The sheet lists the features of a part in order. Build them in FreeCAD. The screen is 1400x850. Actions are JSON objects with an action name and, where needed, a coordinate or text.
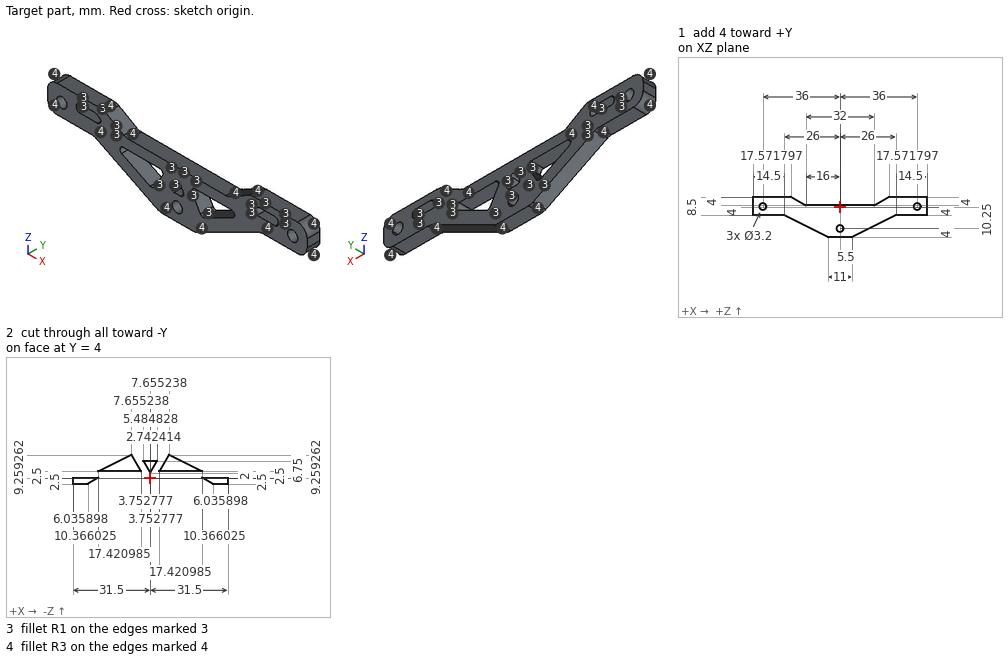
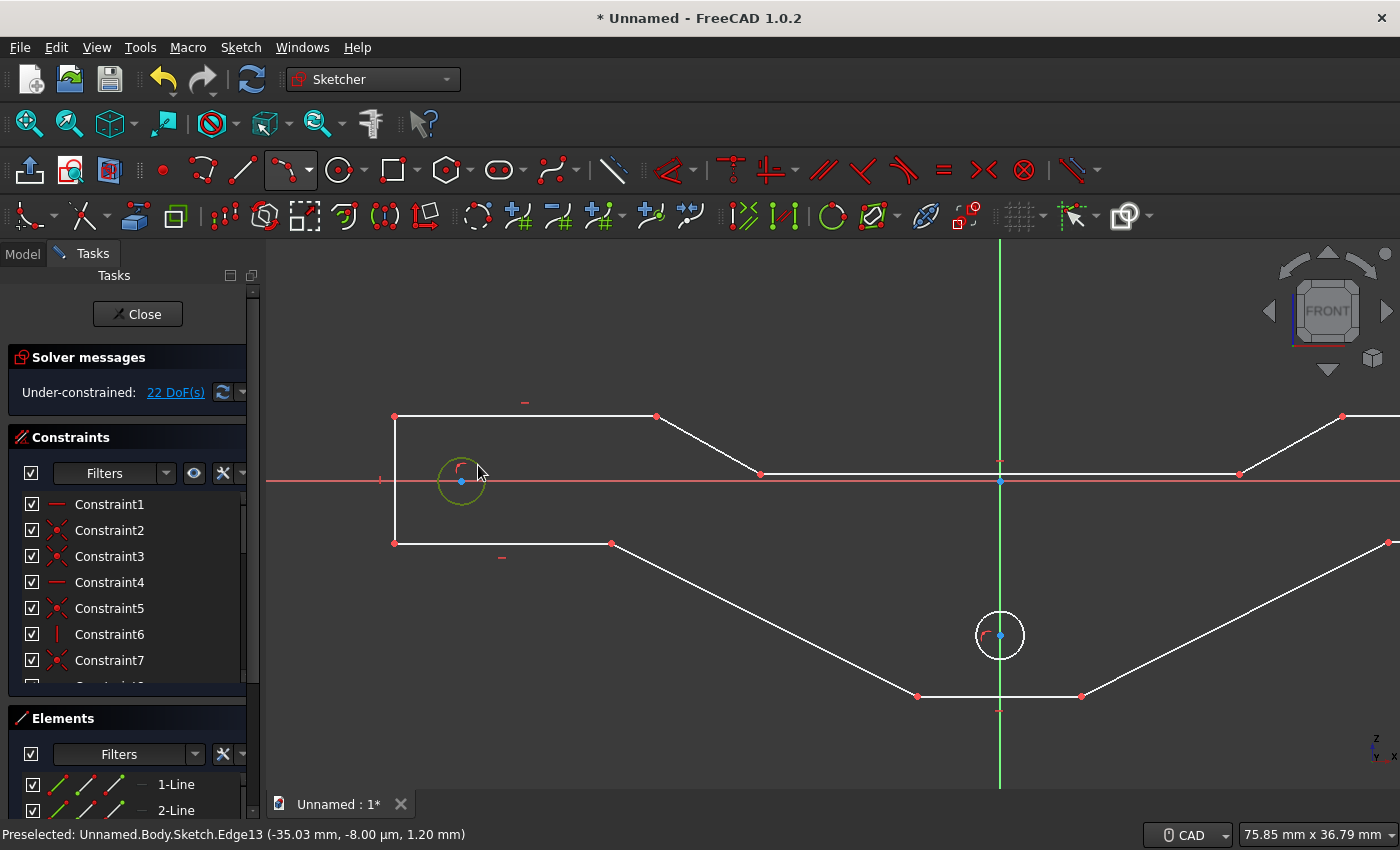
{"action": "scroll", "coordinate": [478, 465], "scroll_direction": "down", "scroll_amount": 3}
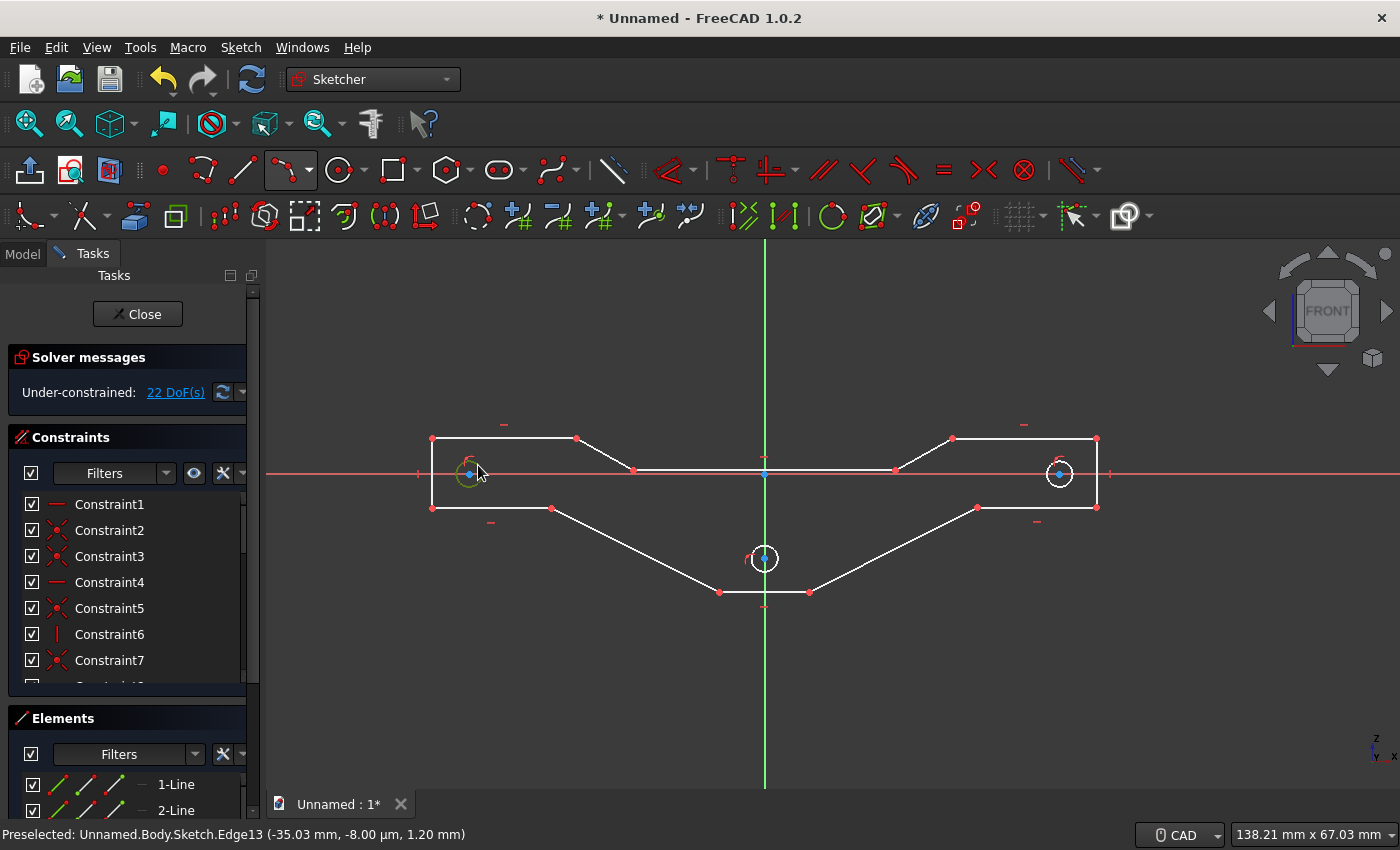
{"action": "scroll", "coordinate": [1069, 465], "scroll_direction": "up", "scroll_amount": 3}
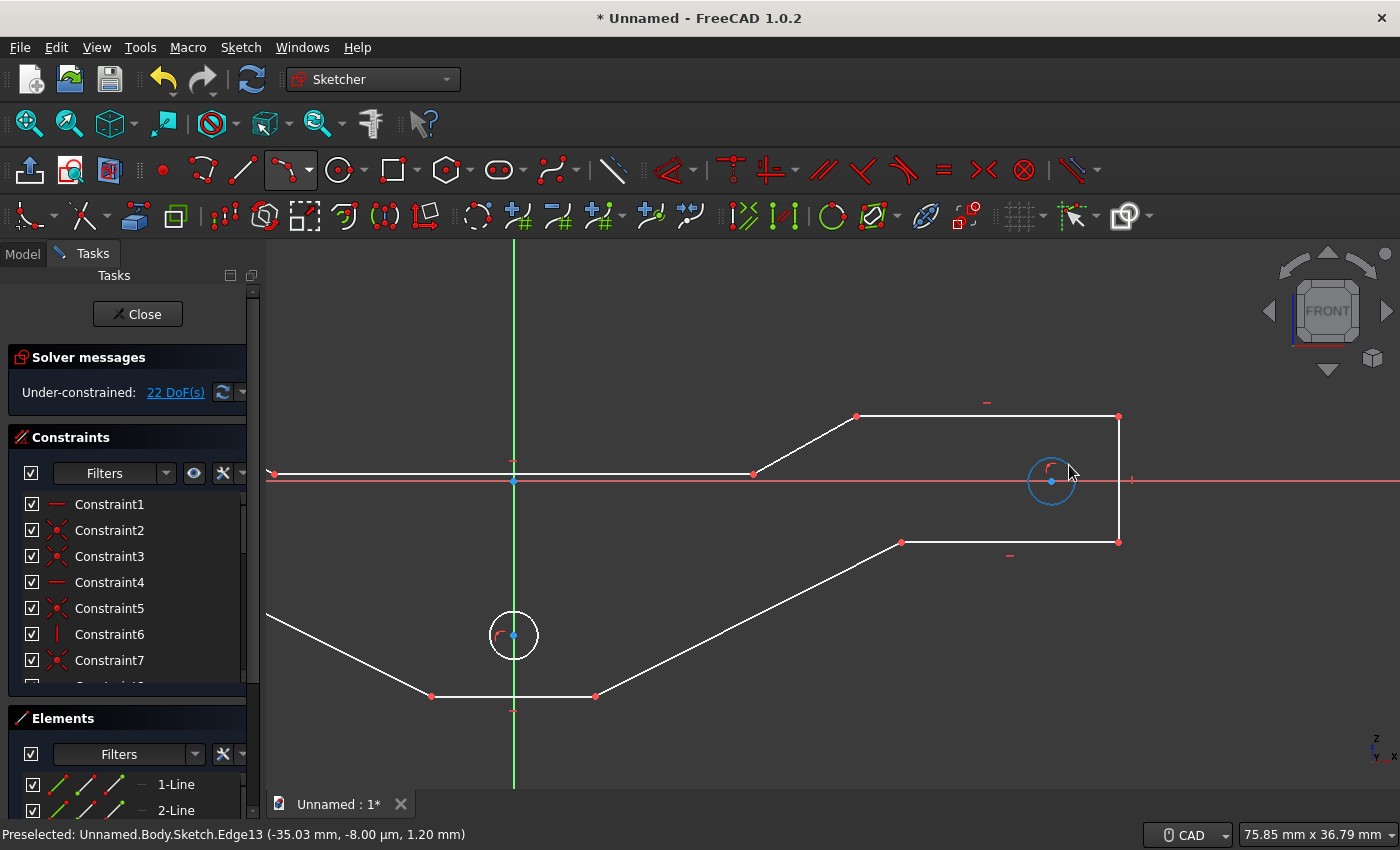
{"action": "left_click", "coordinate": [1068, 465]}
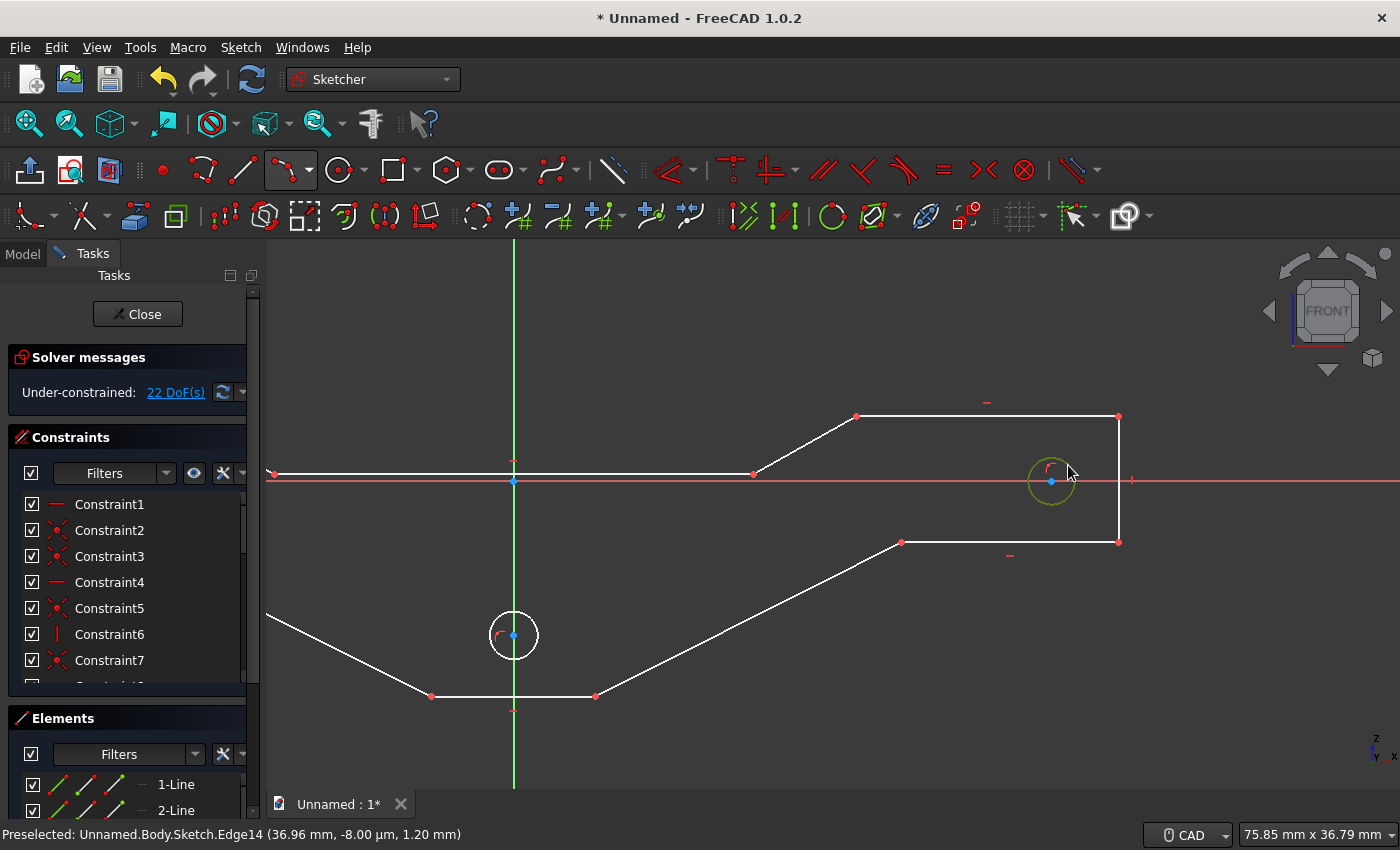
{"action": "left_click", "coordinate": [531, 618]}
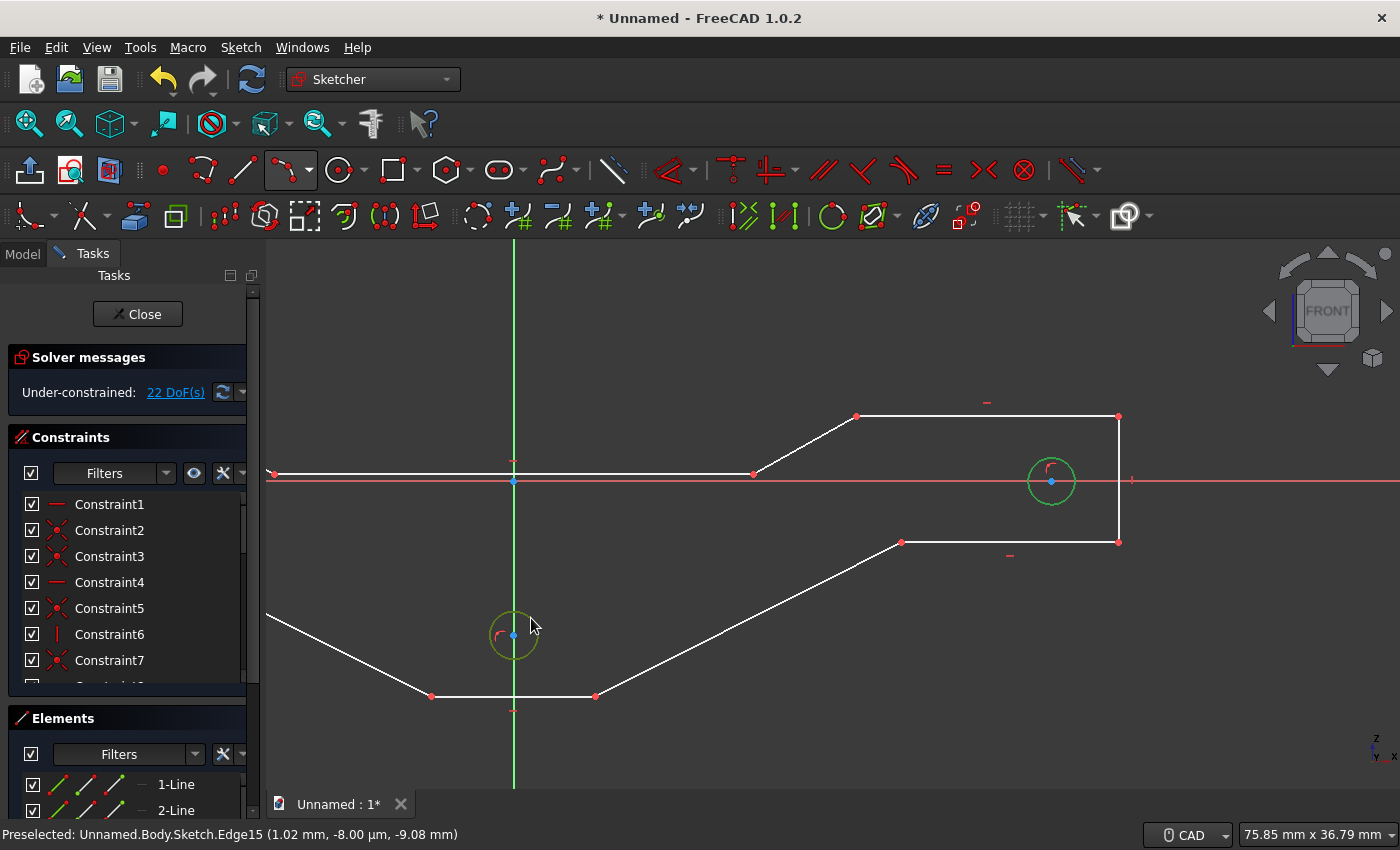
{"action": "left_click", "coordinate": [944, 170]}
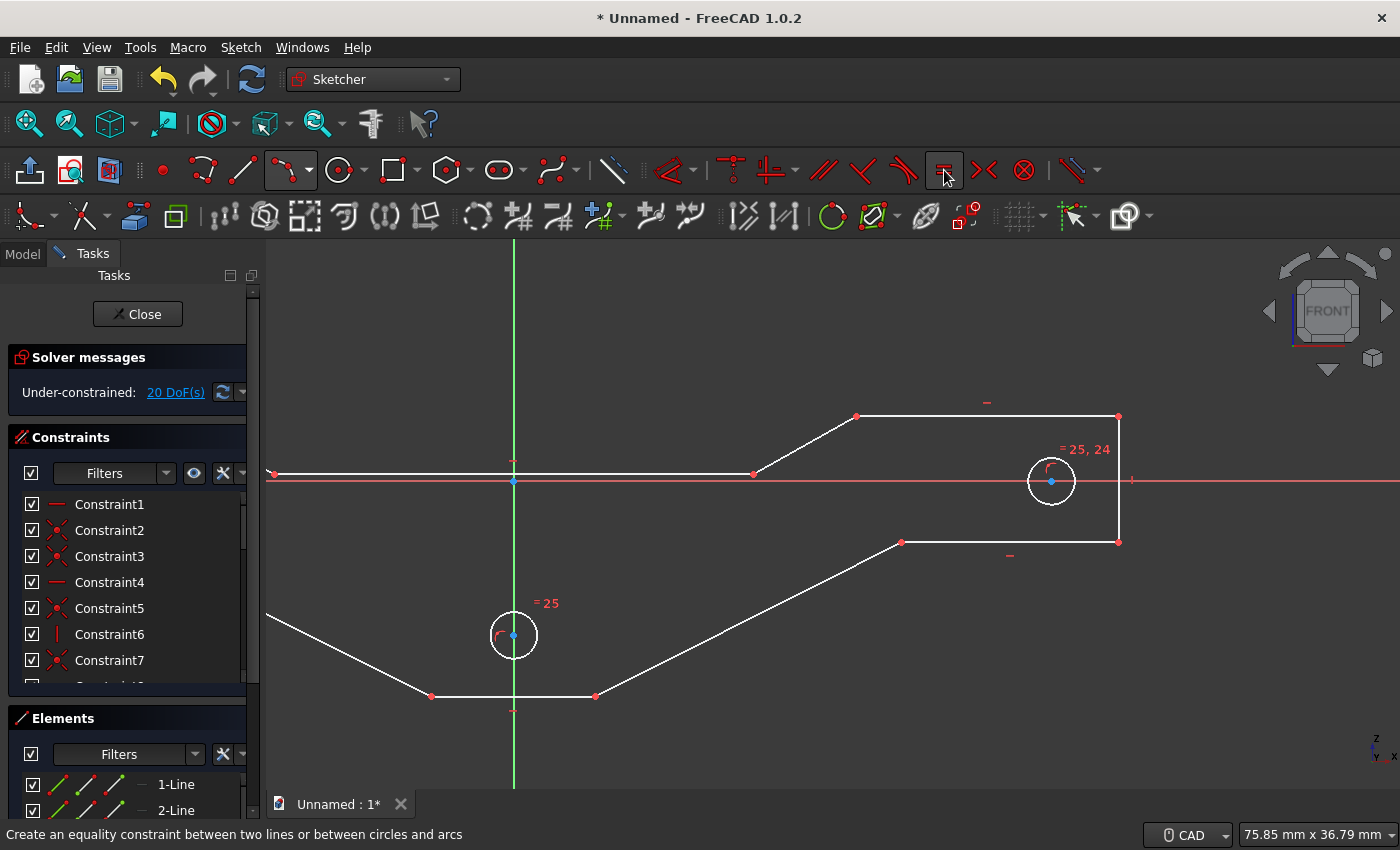
{"action": "left_click", "coordinate": [668, 170]}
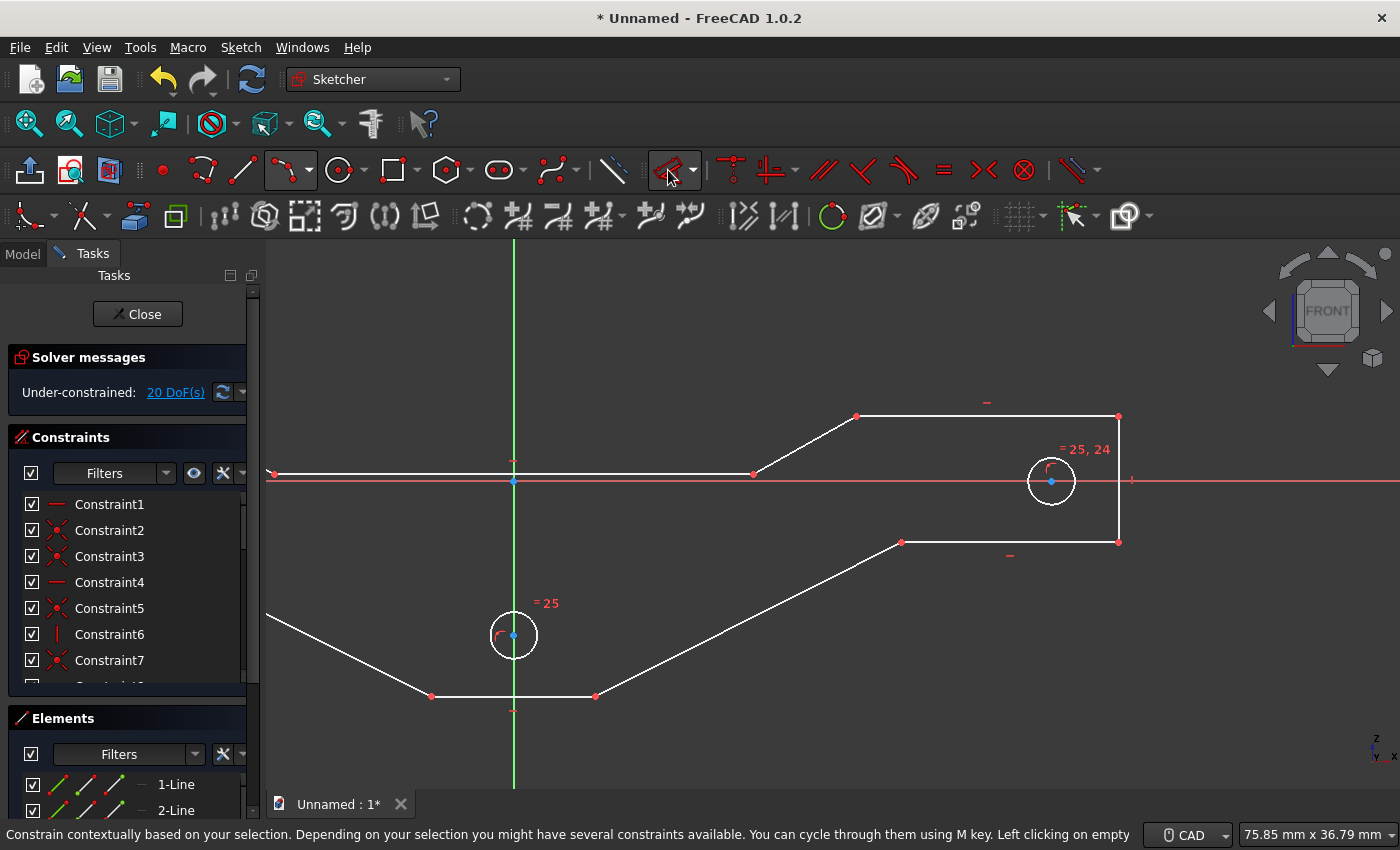
{"action": "scroll", "coordinate": [1069, 465], "scroll_direction": "down", "scroll_amount": 3}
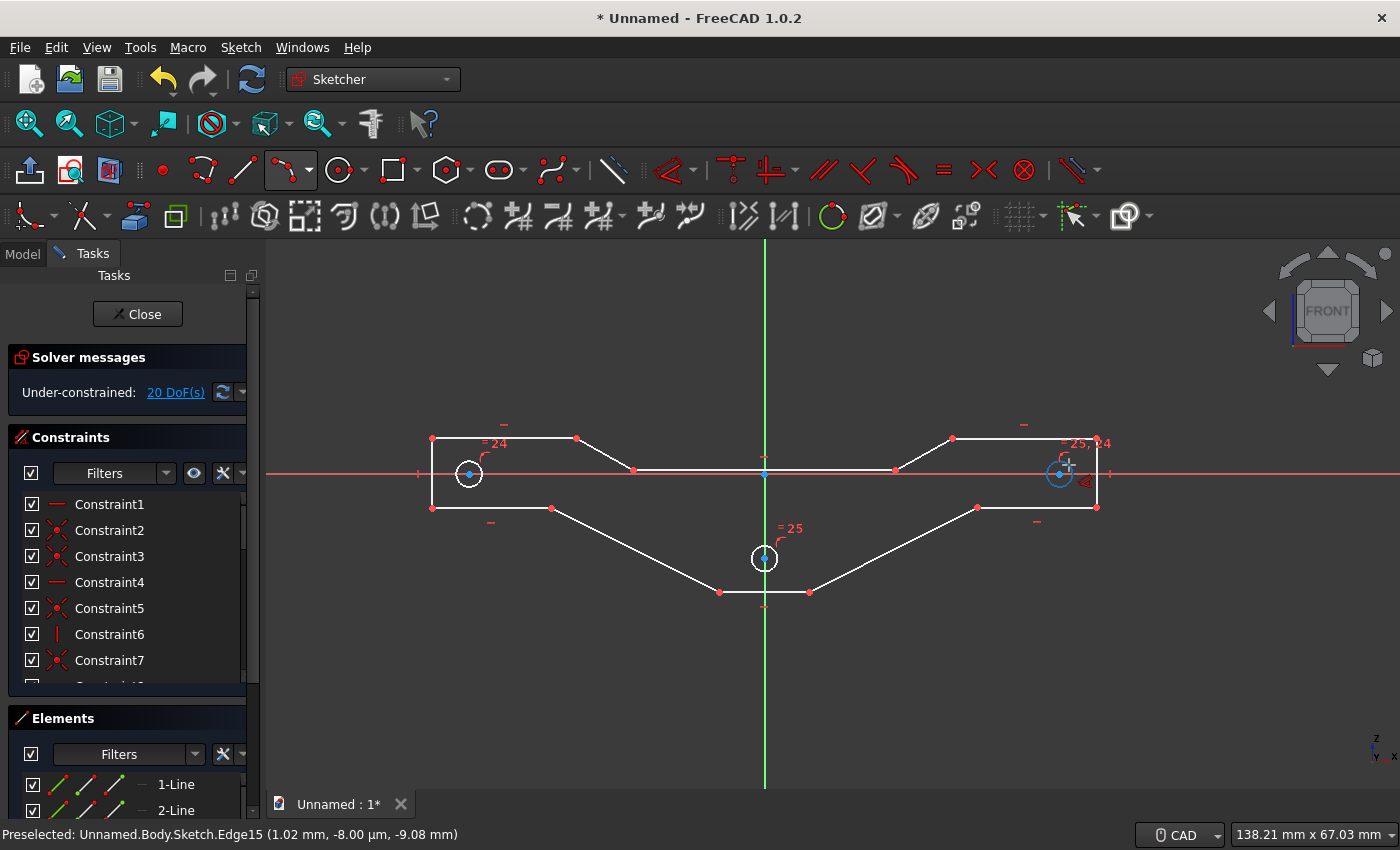
{"action": "scroll", "coordinate": [478, 465], "scroll_direction": "up", "scroll_amount": 3}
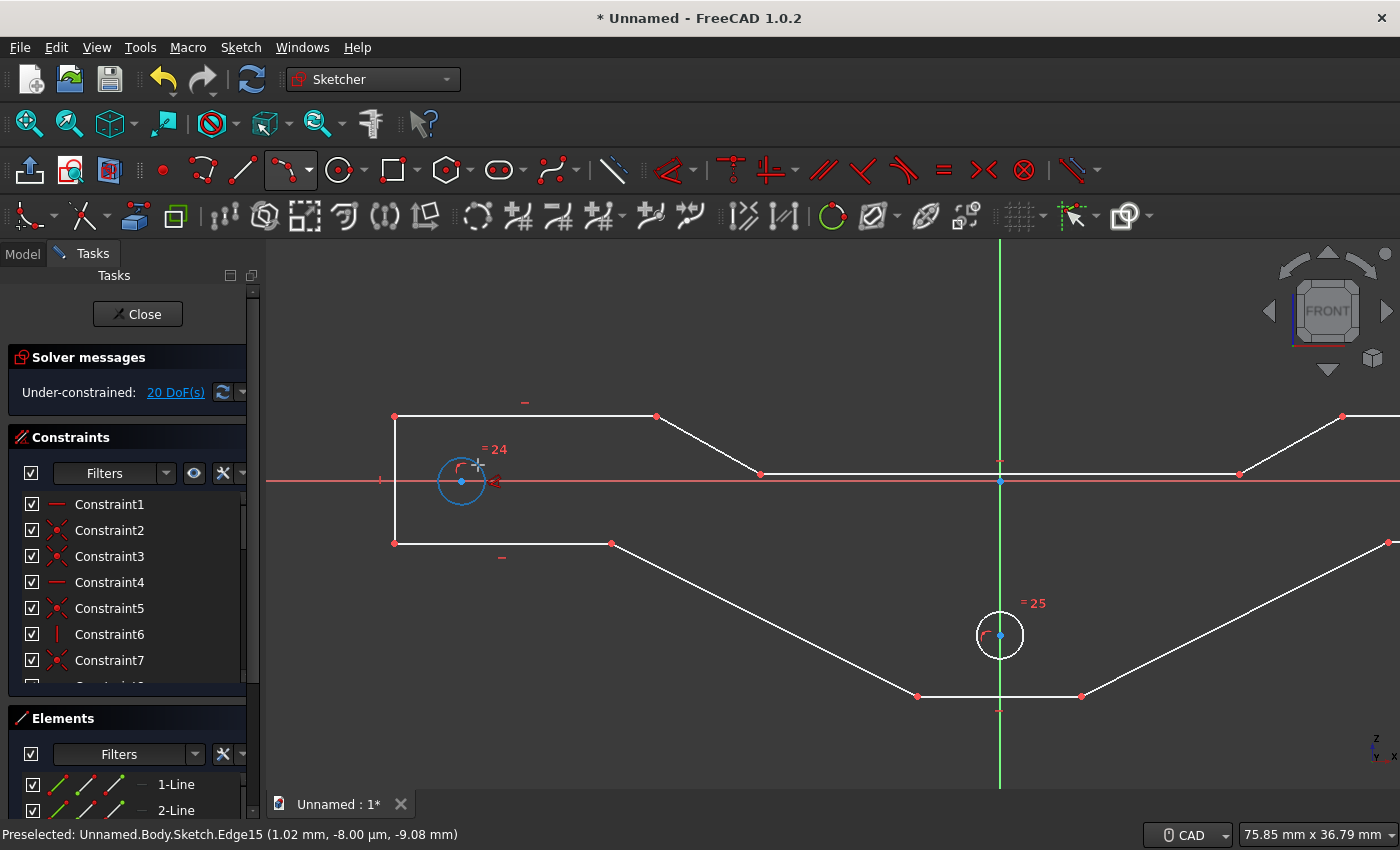
{"action": "left_click", "coordinate": [478, 465]}
{"action": "left_click", "coordinate": [501, 442]}